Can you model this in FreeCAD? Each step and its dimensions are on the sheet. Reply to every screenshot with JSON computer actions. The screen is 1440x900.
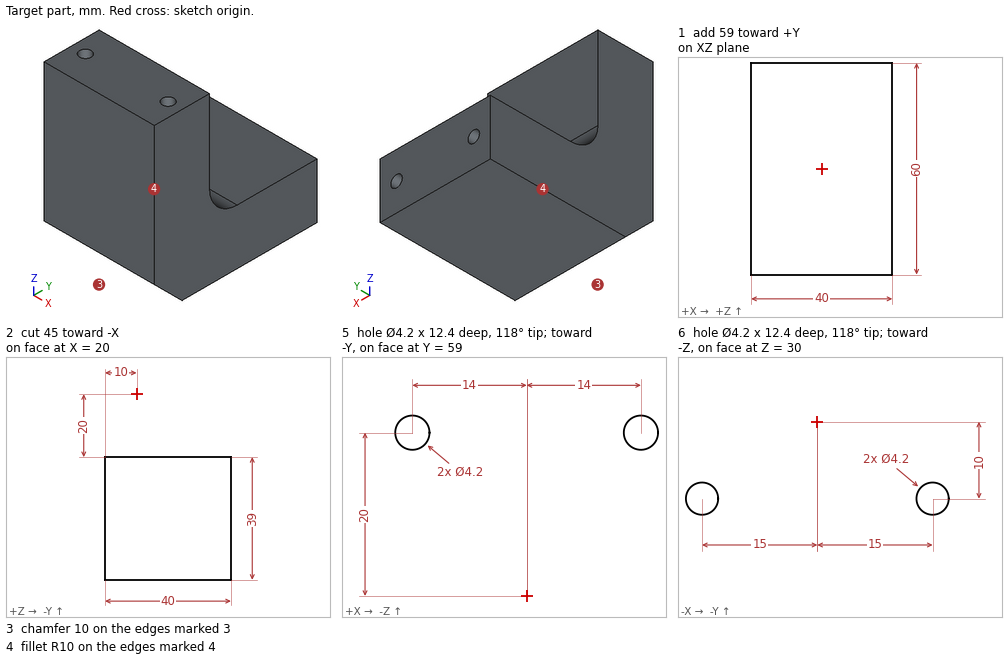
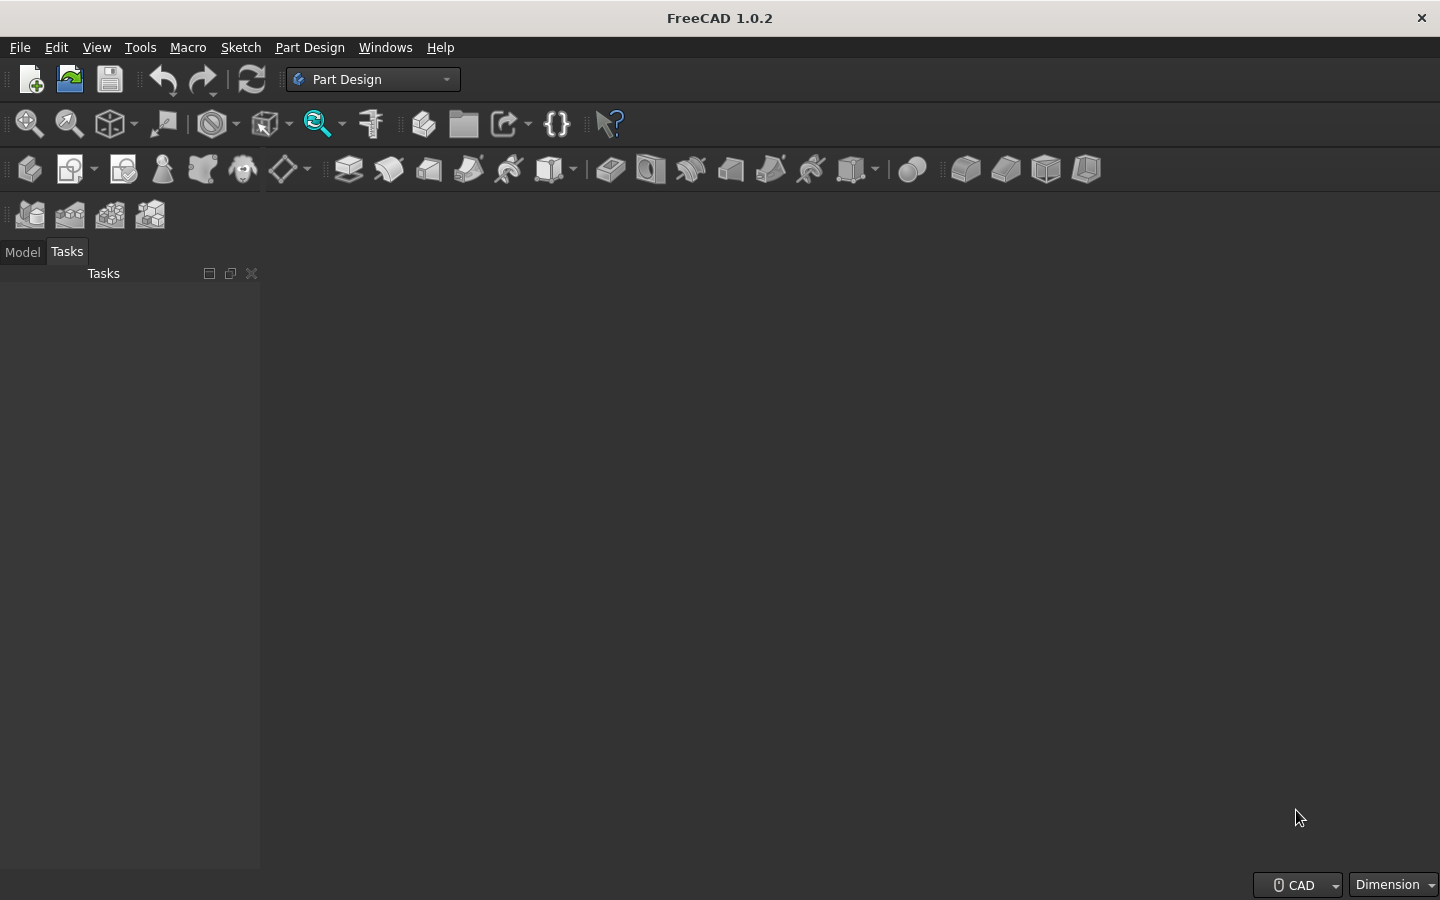
{"action": "left_click", "coordinate": [30, 80]}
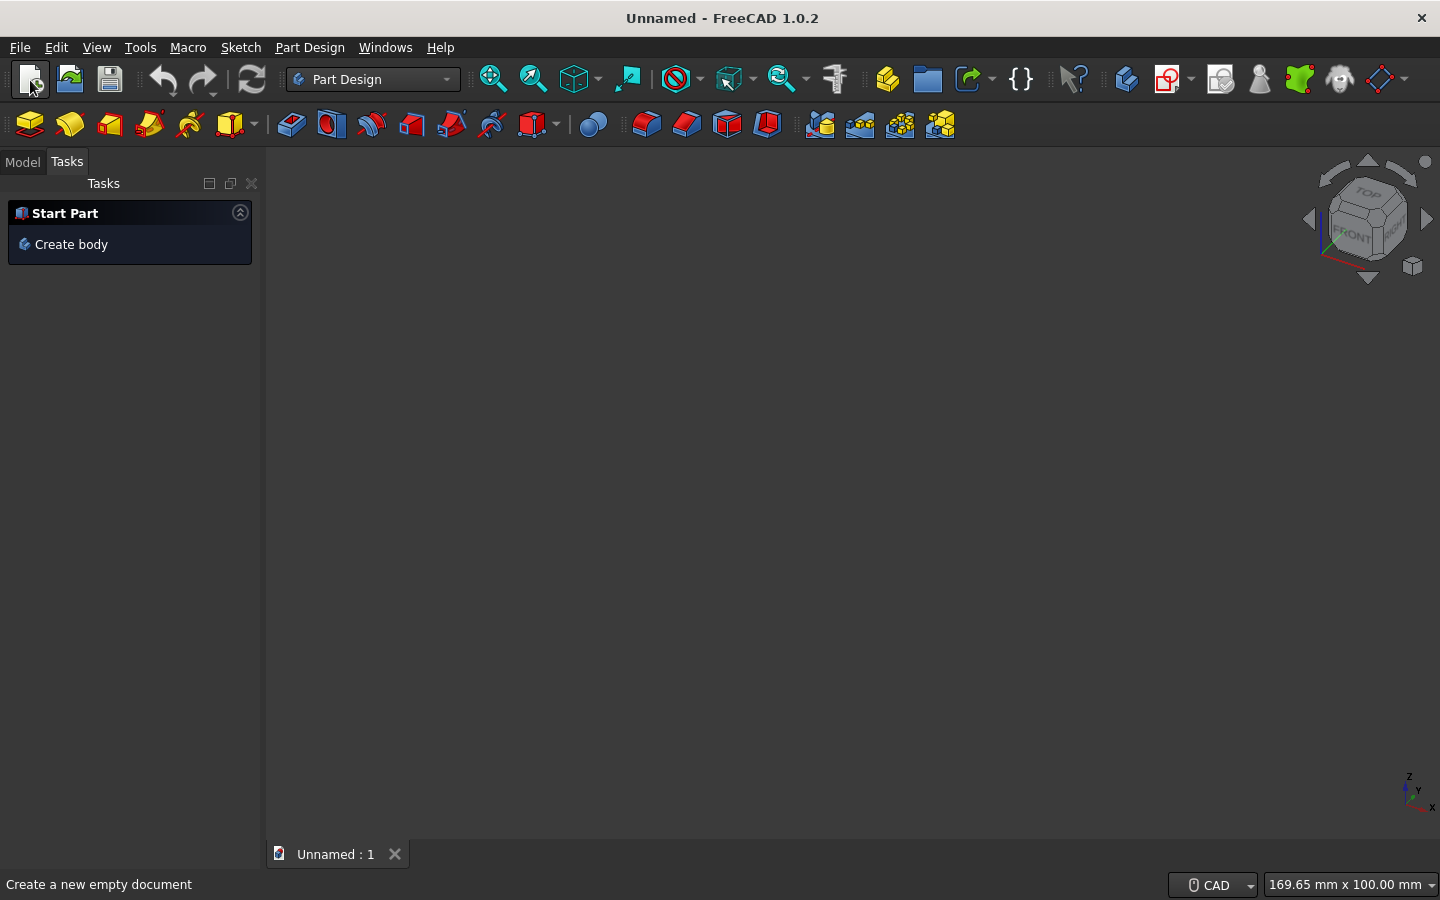
{"action": "left_click", "coordinate": [1168, 80]}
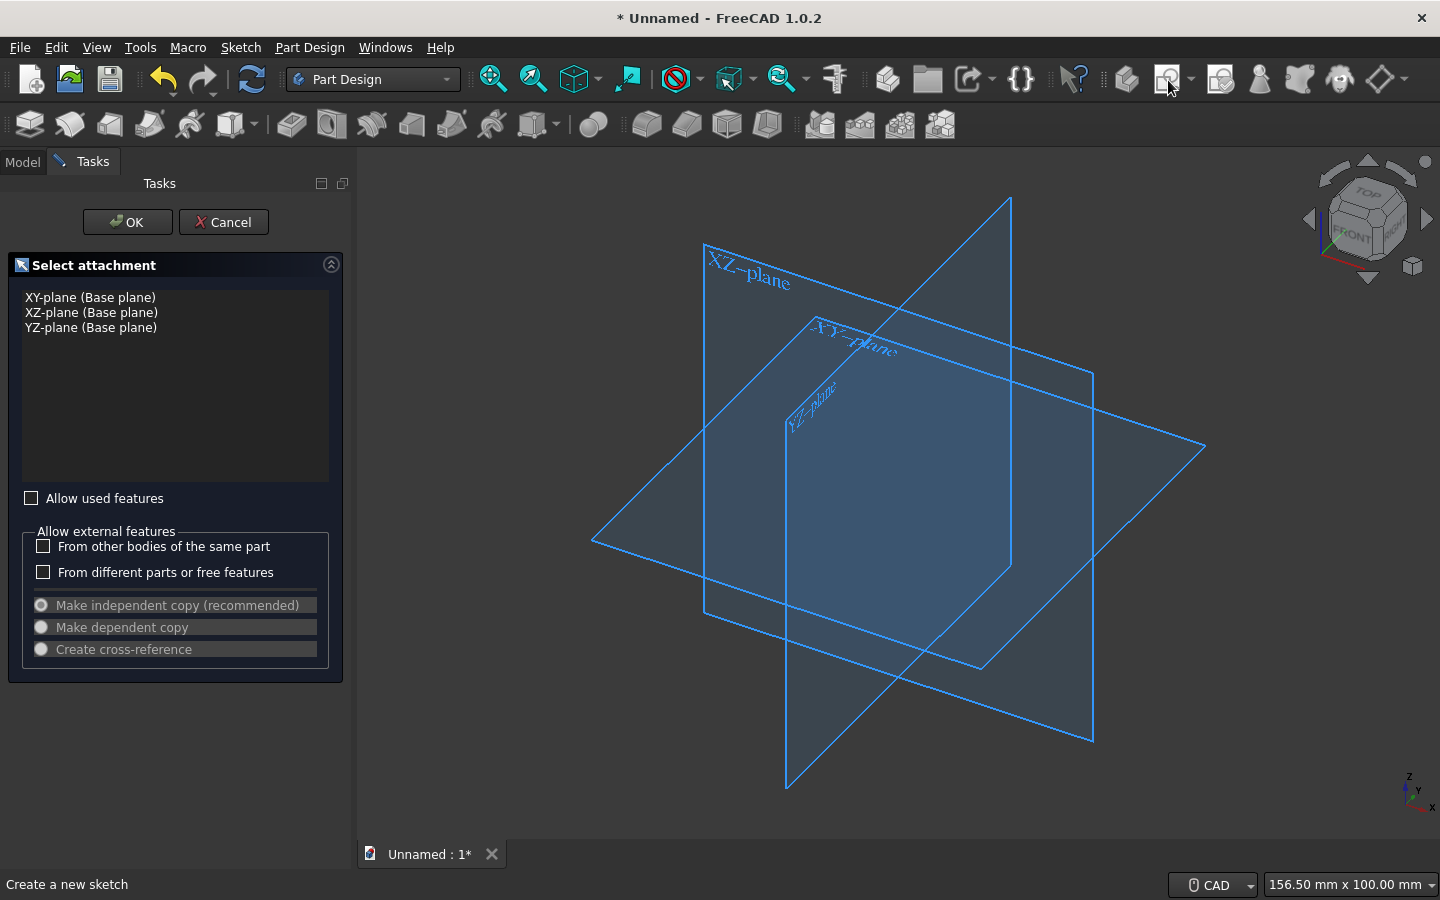
{"action": "left_click", "coordinate": [82, 312]}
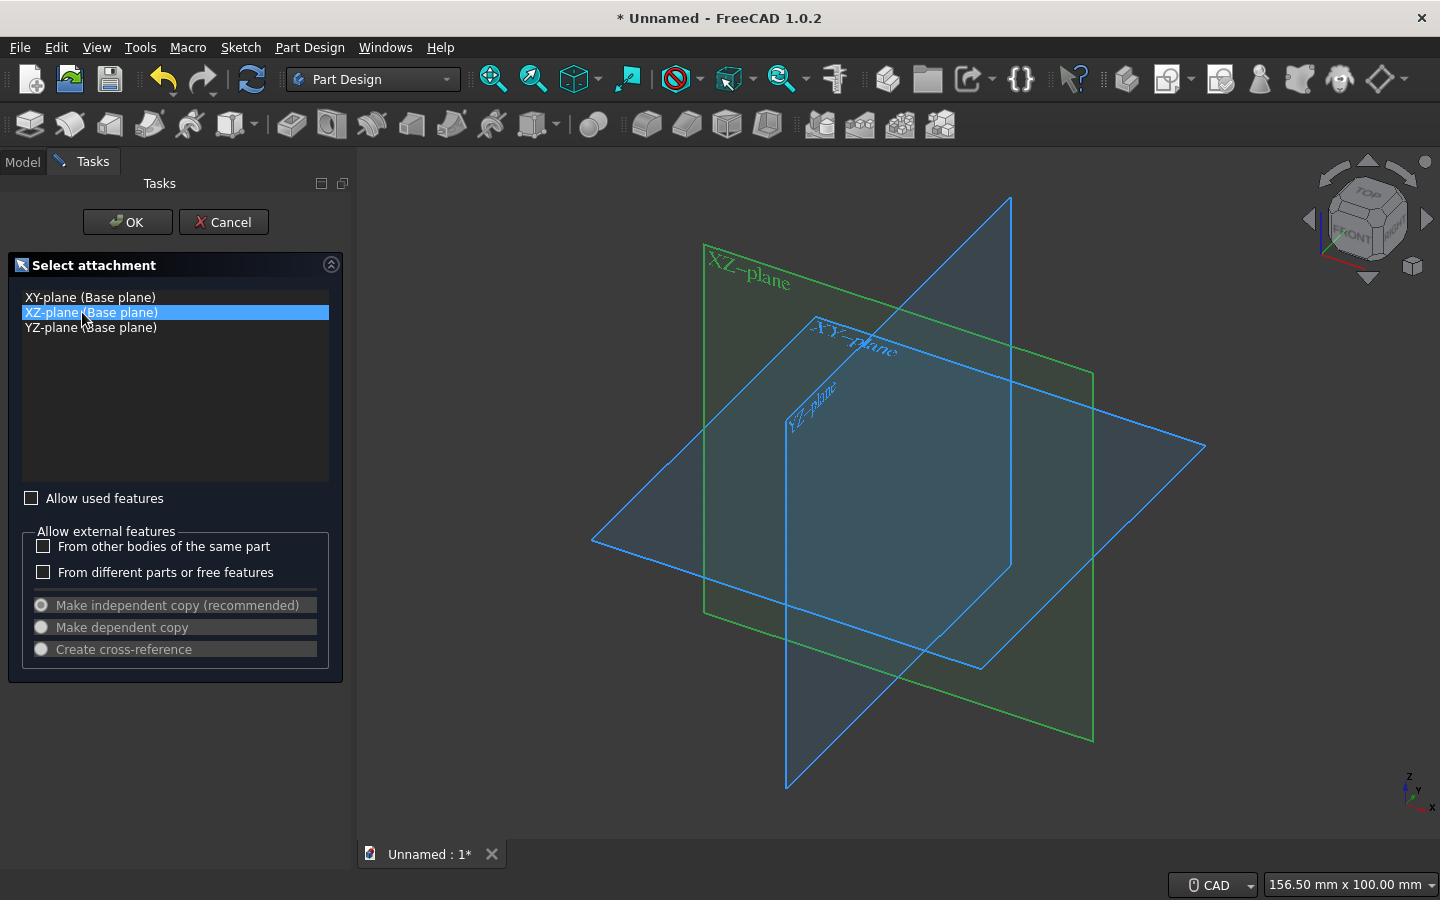
{"action": "left_click", "coordinate": [128, 222]}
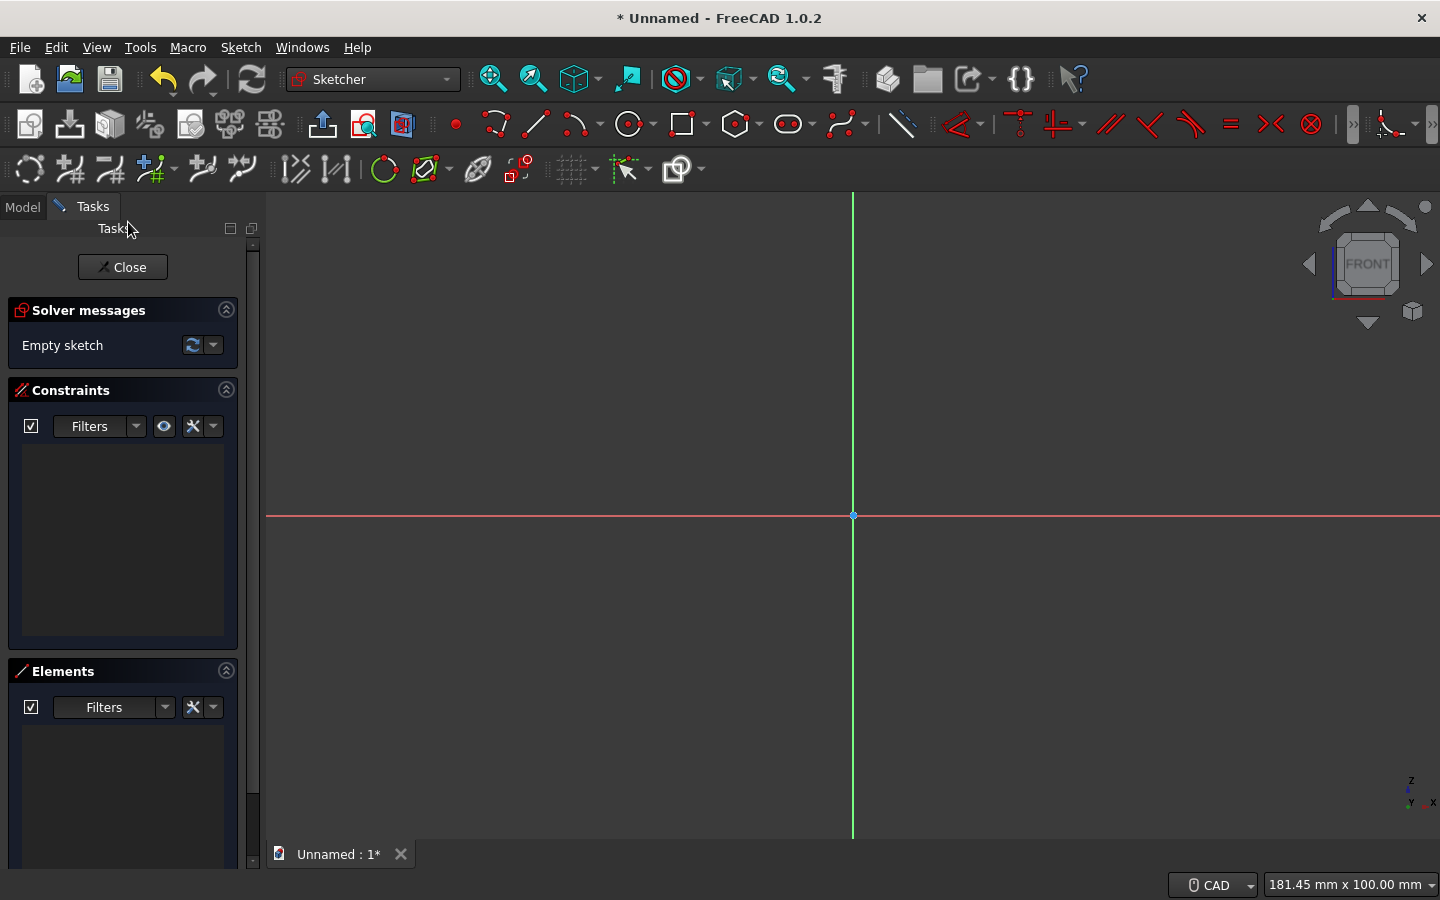
{"action": "key", "text": "g v"}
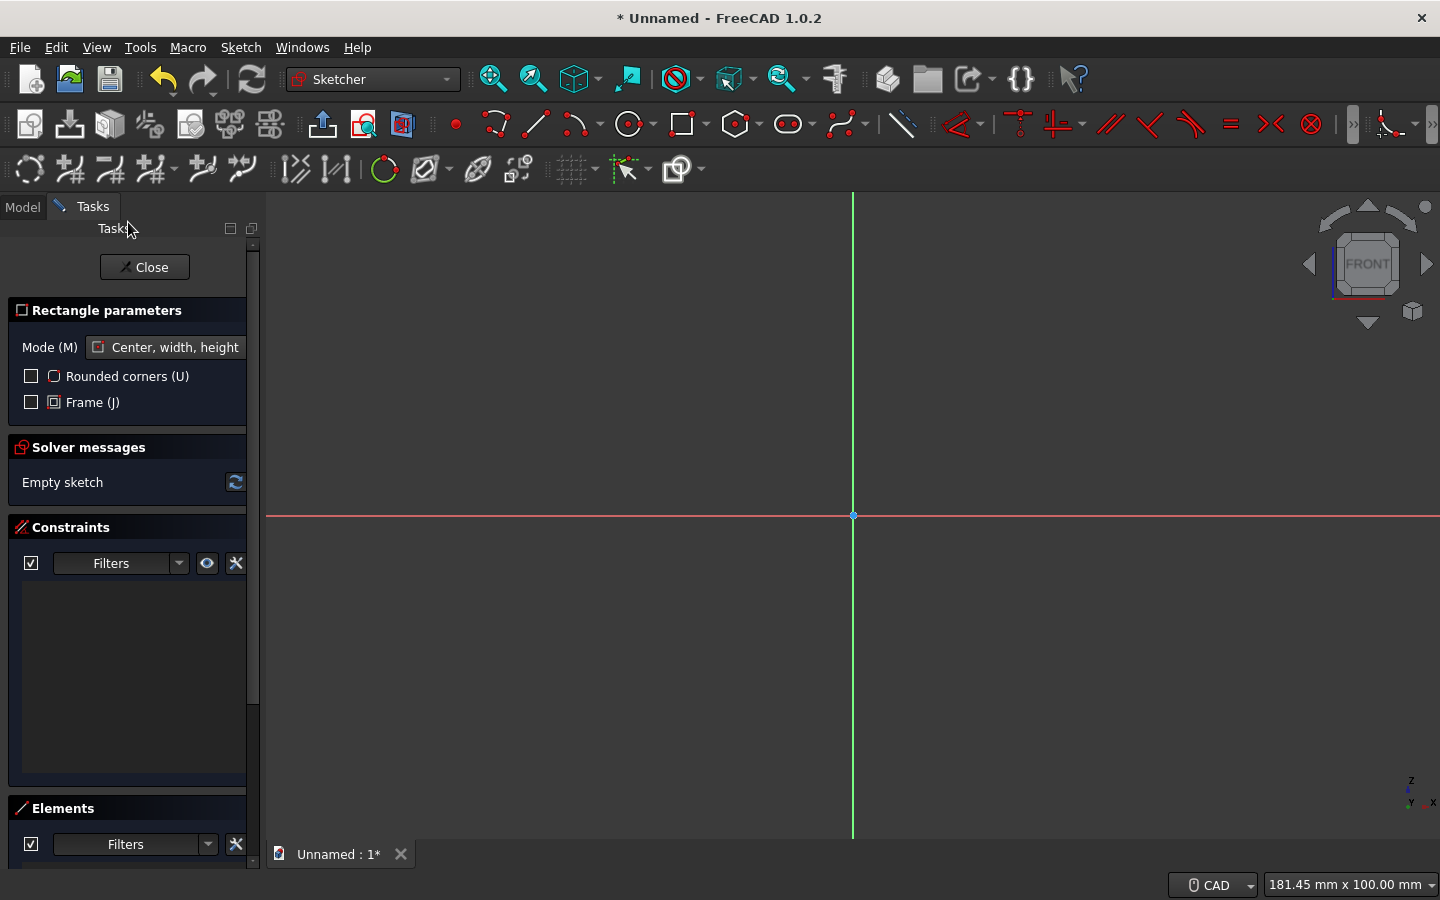
{"action": "left_click", "coordinate": [853, 516]}
{"action": "mouse_move", "coordinate": [982, 321]}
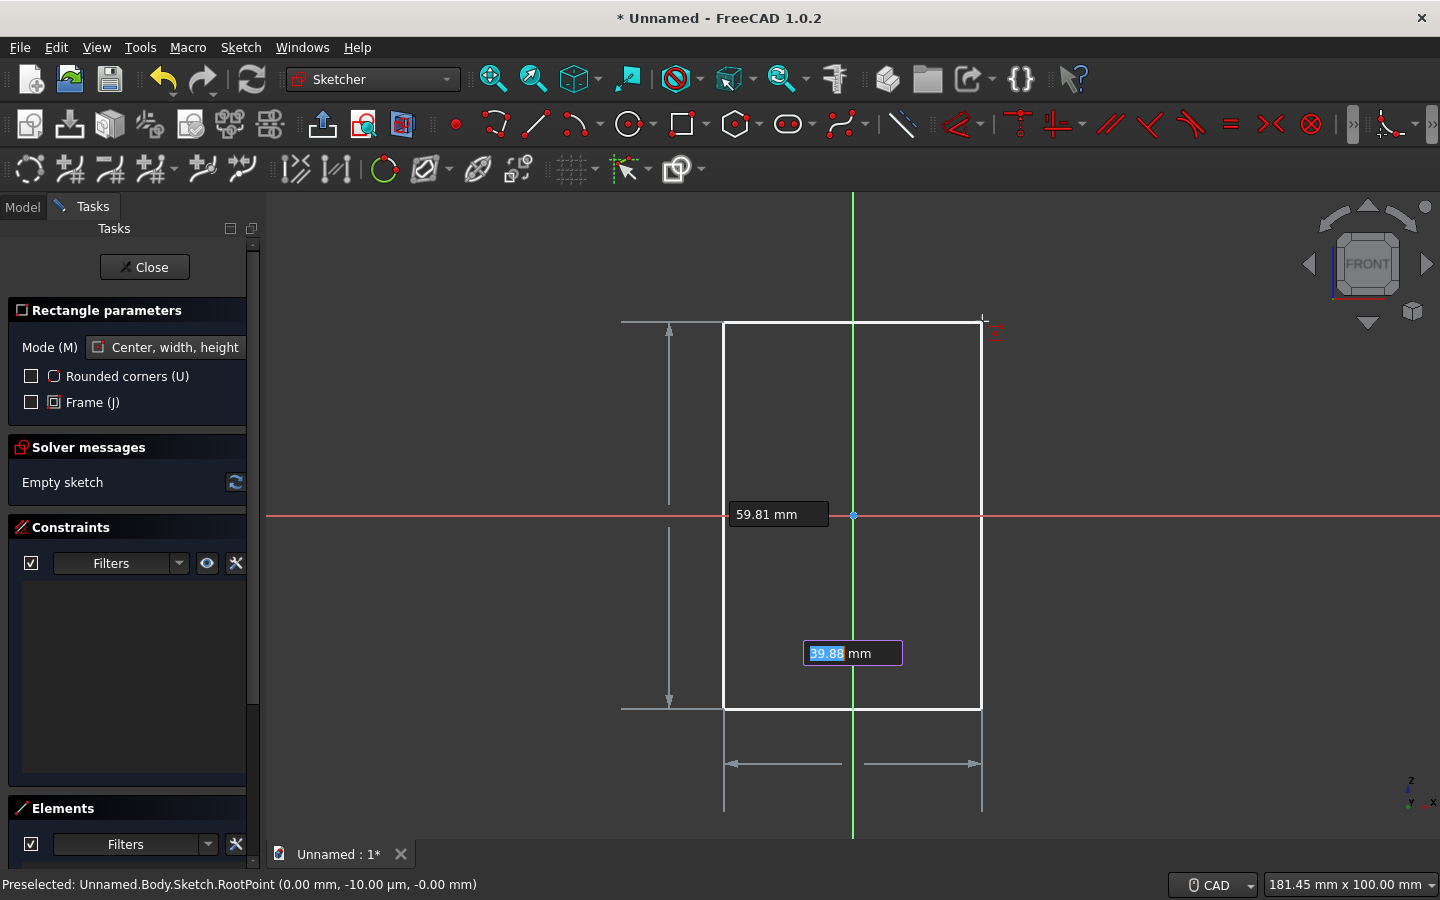
{"action": "type", "text": "40"}
{"action": "key", "text": "Tab"}
{"action": "type", "text": "60"}
{"action": "key", "text": "Return"}
{"action": "key", "text": "Escape"}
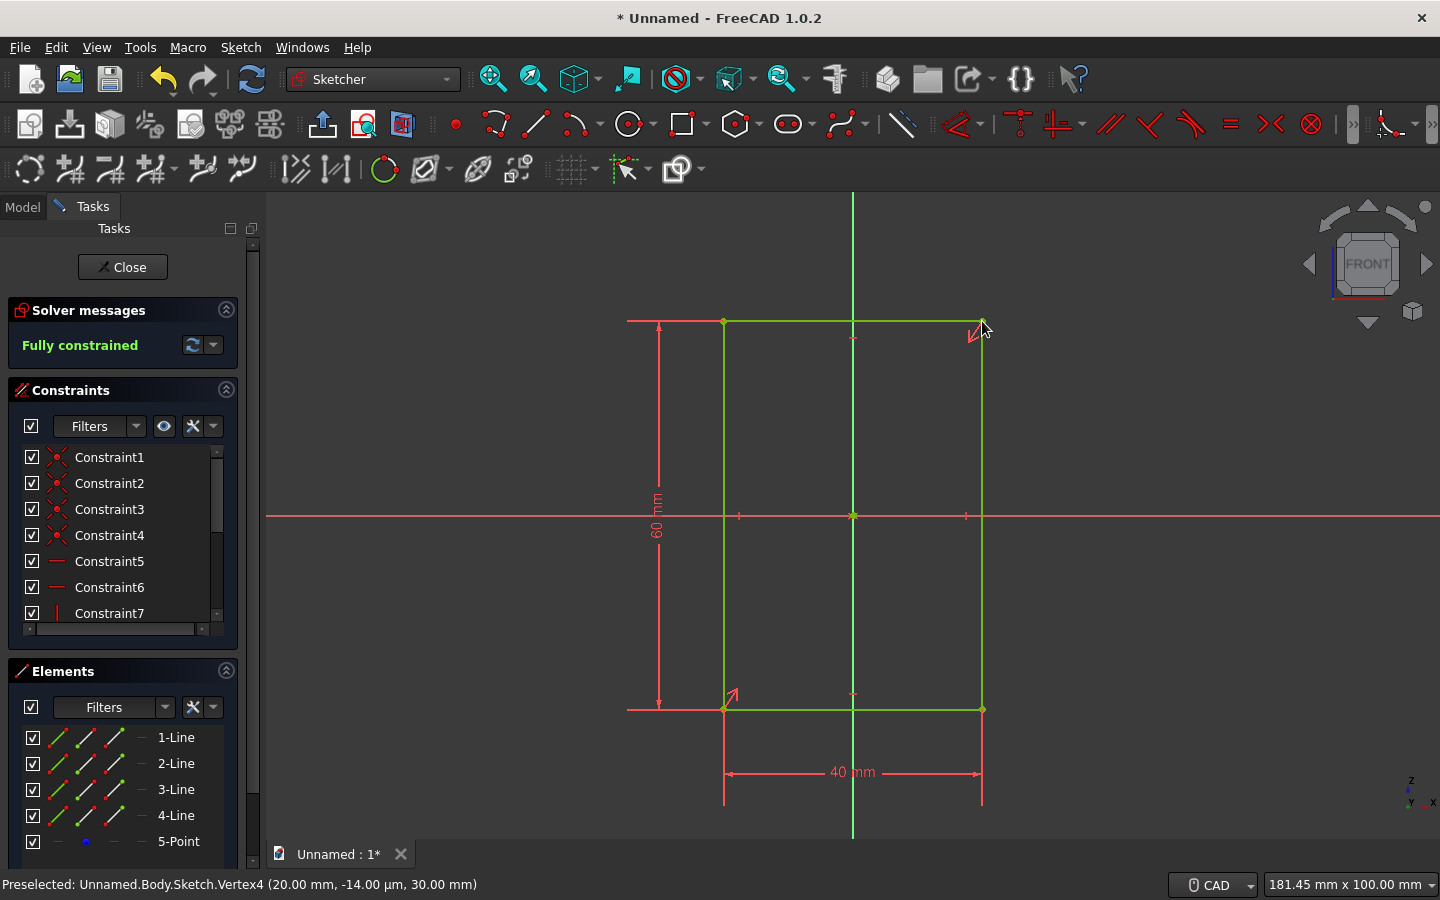
{"action": "left_click", "coordinate": [123, 267]}